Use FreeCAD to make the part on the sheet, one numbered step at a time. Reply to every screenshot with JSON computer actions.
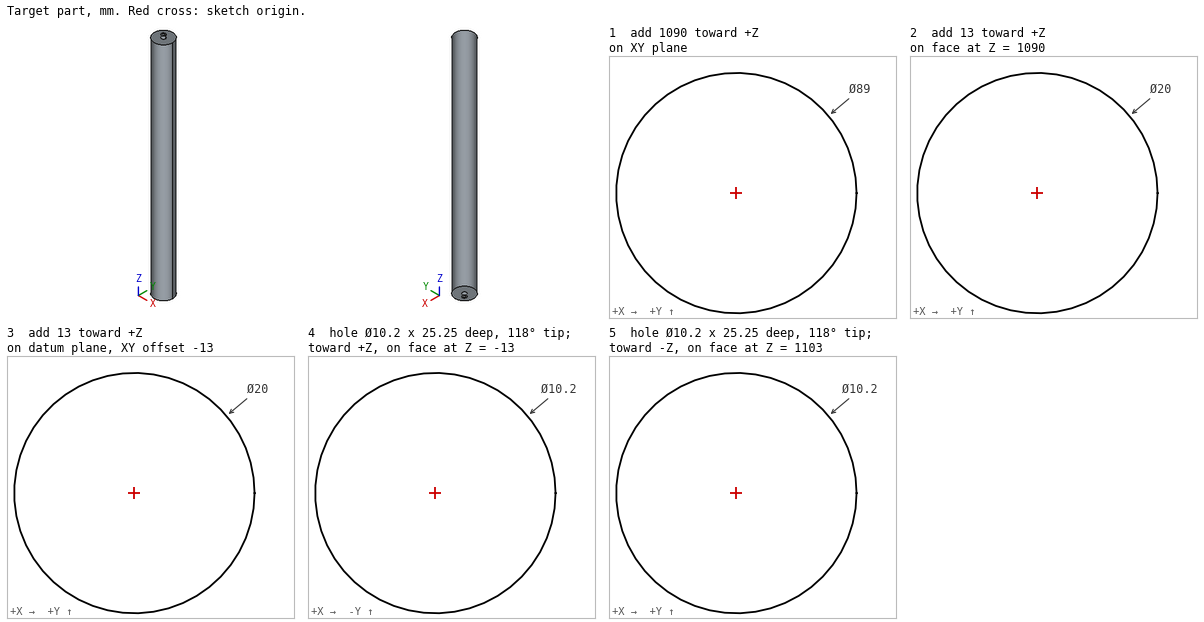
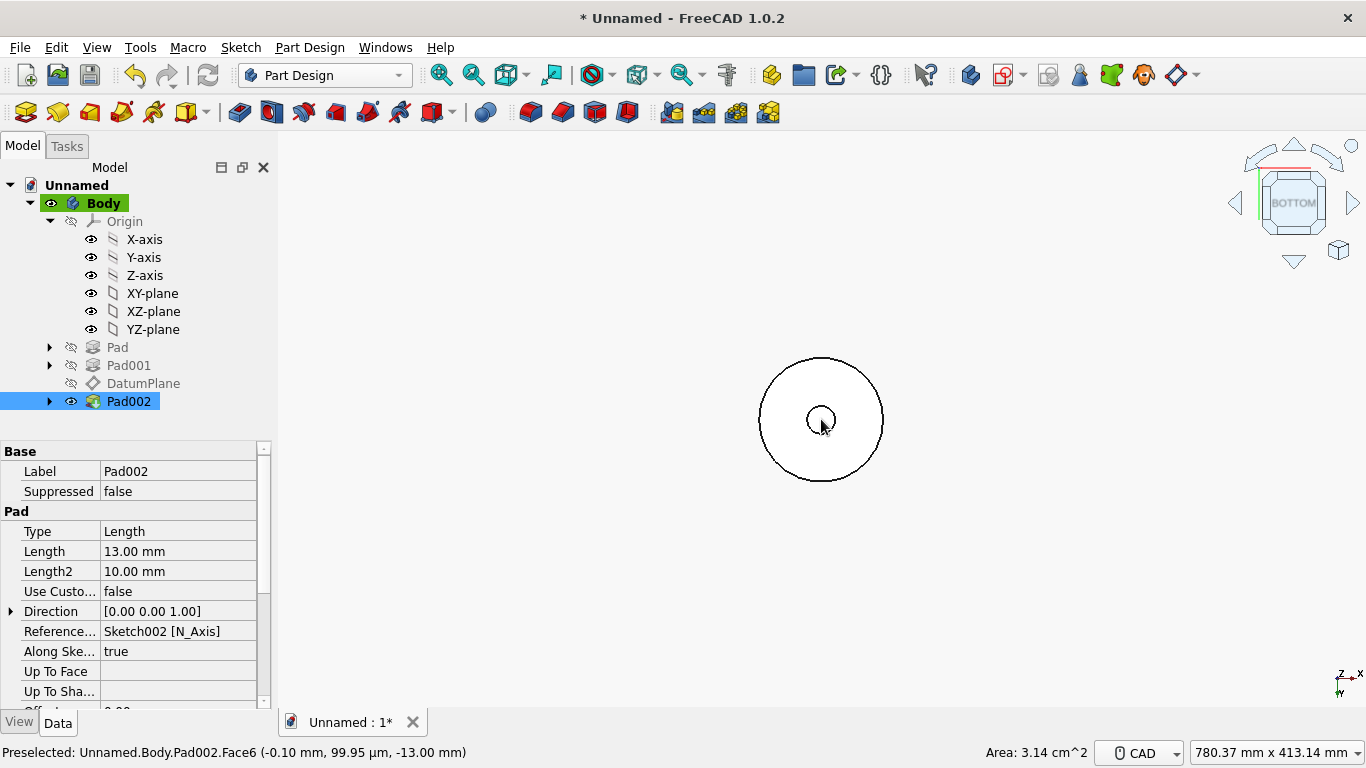
{"action": "left_click", "coordinate": [1004, 76]}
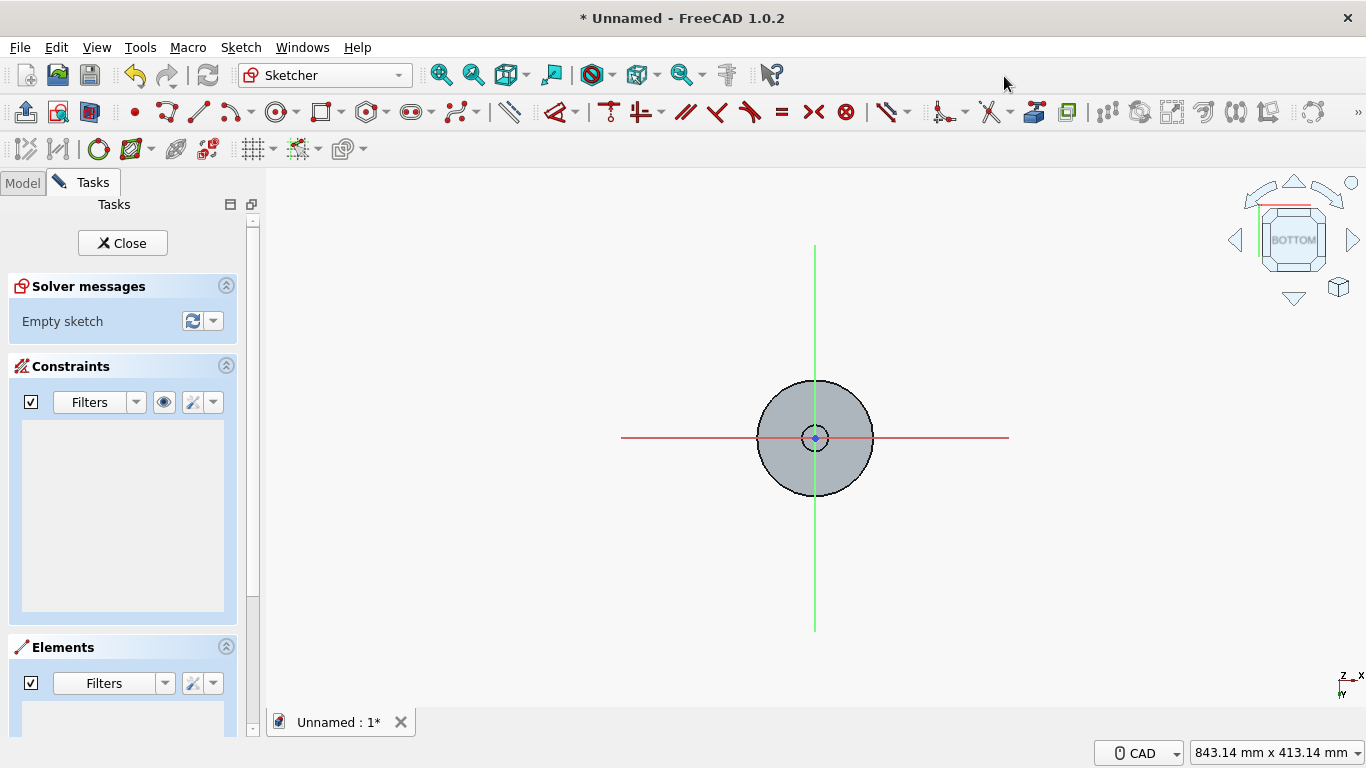
{"action": "scroll", "coordinate": [819, 438], "scroll_direction": "up", "scroll_amount": 15}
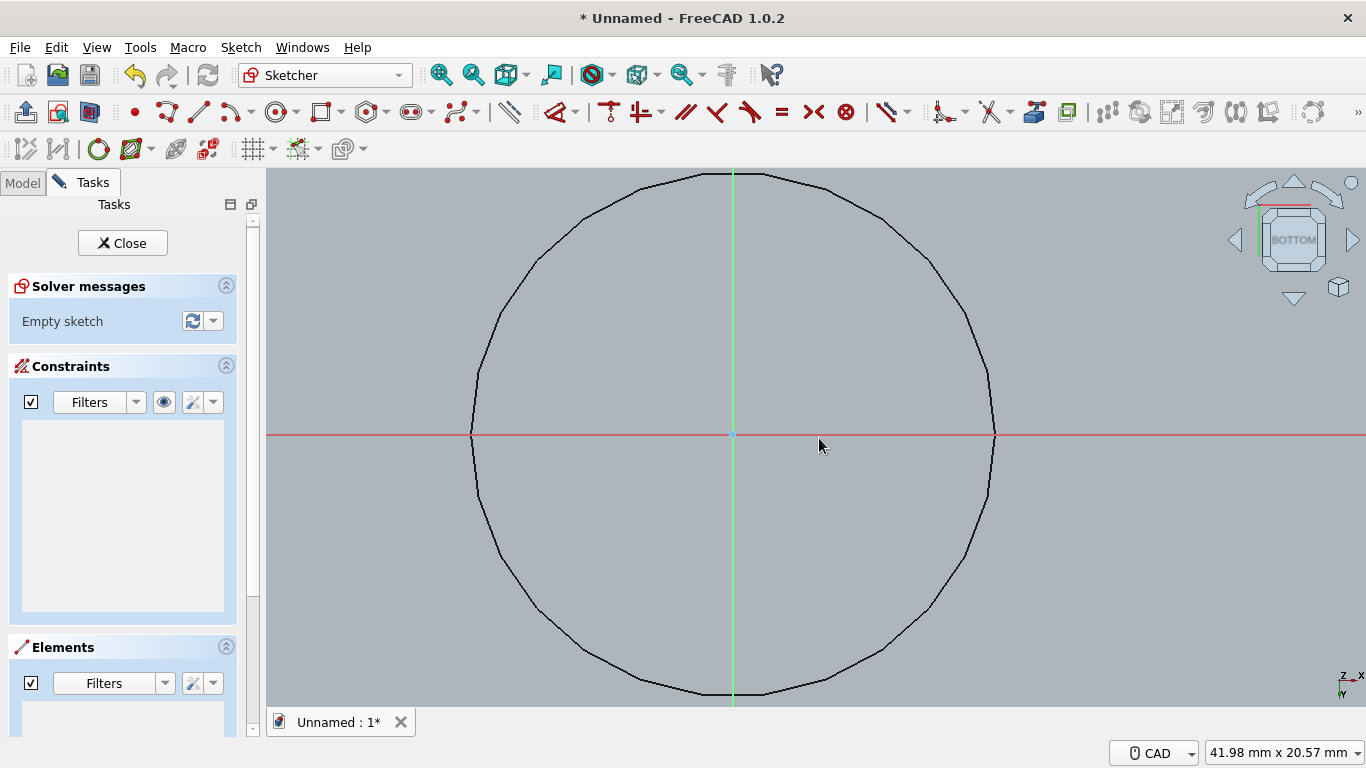
{"action": "key", "text": "g c"}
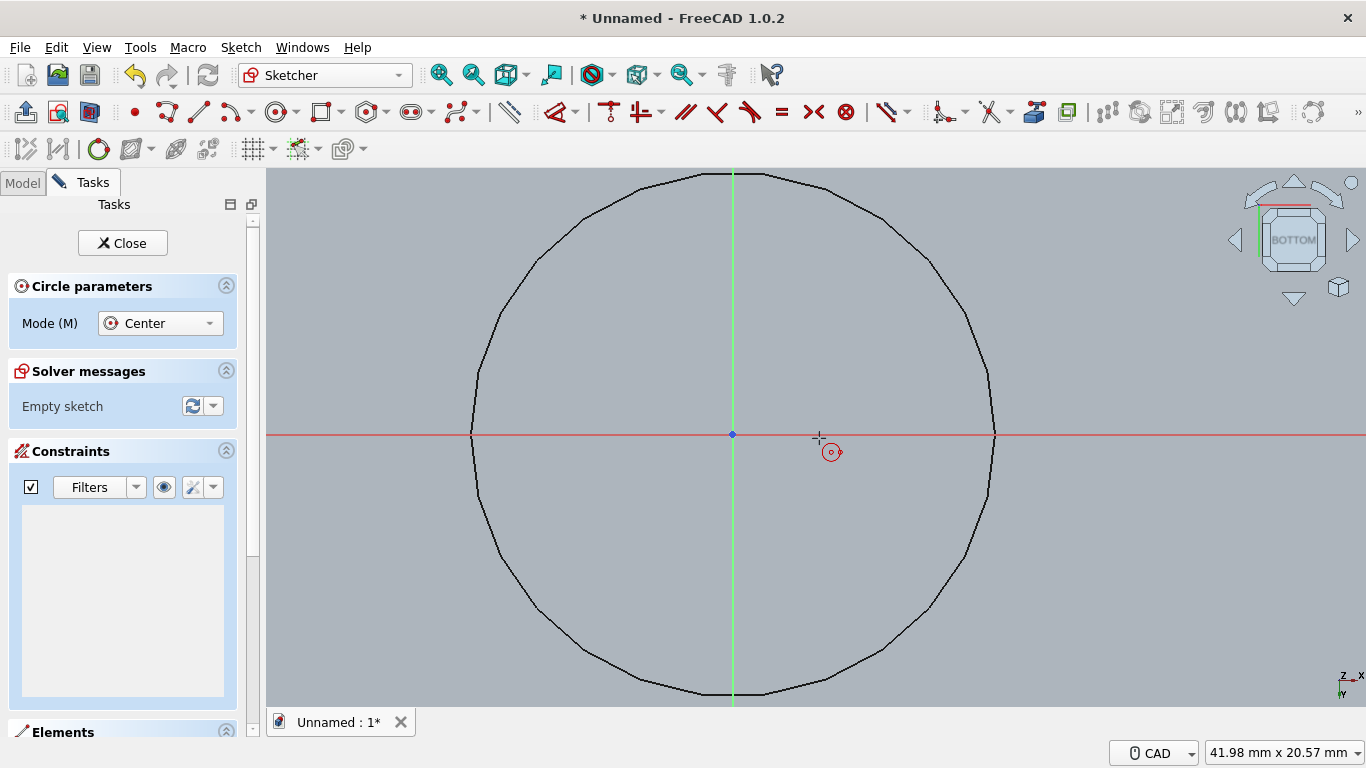
{"action": "left_click", "coordinate": [733, 435]}
{"action": "mouse_move", "coordinate": [827, 340]}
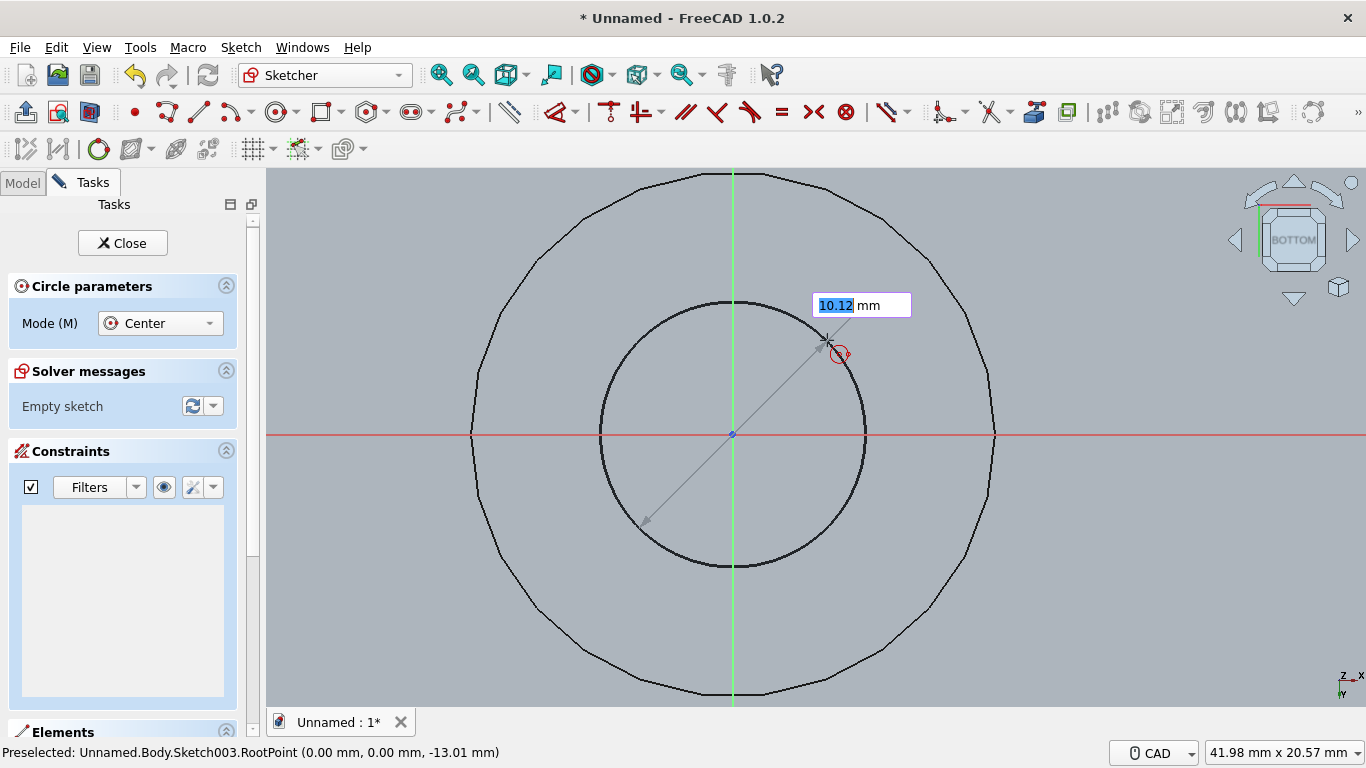
{"action": "type", "text": "10.2"}
{"action": "key", "text": "Return"}
{"action": "key", "text": "Escape"}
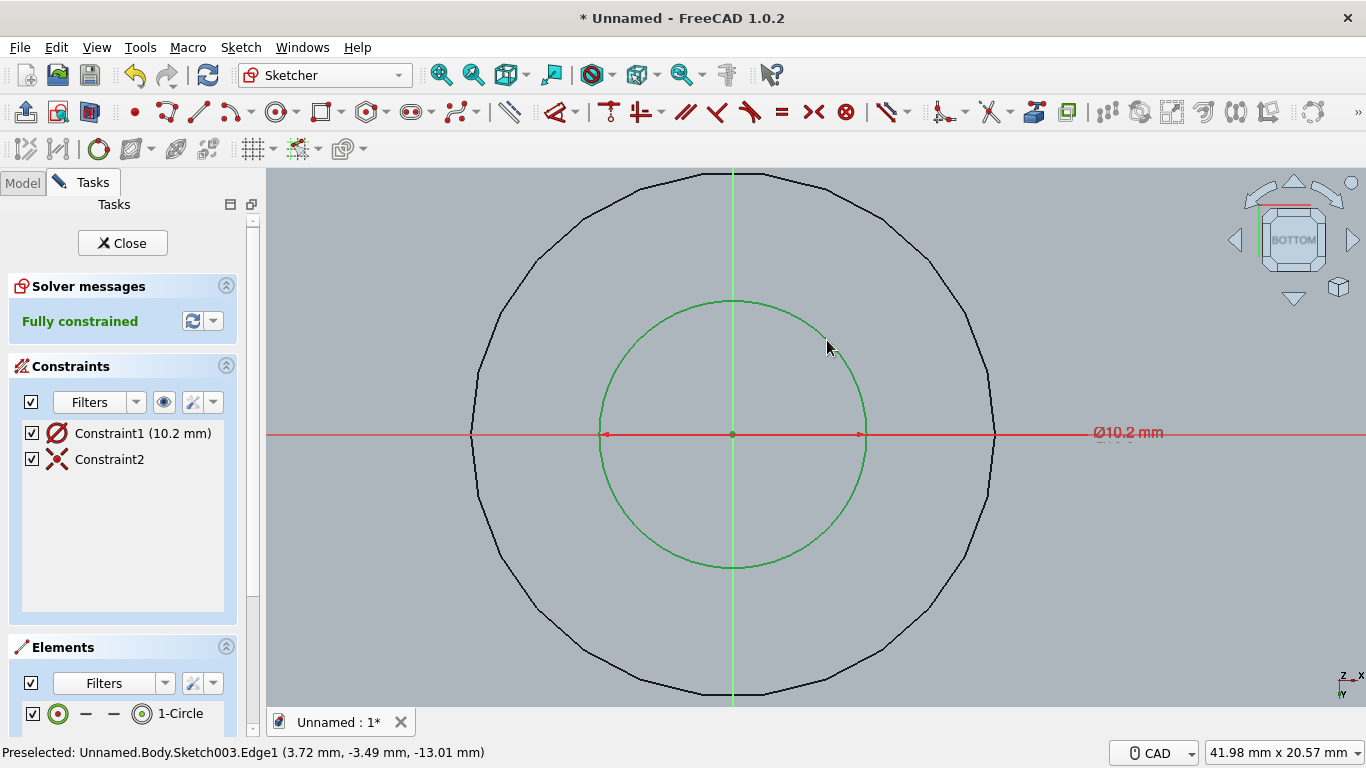
{"action": "left_click", "coordinate": [123, 243]}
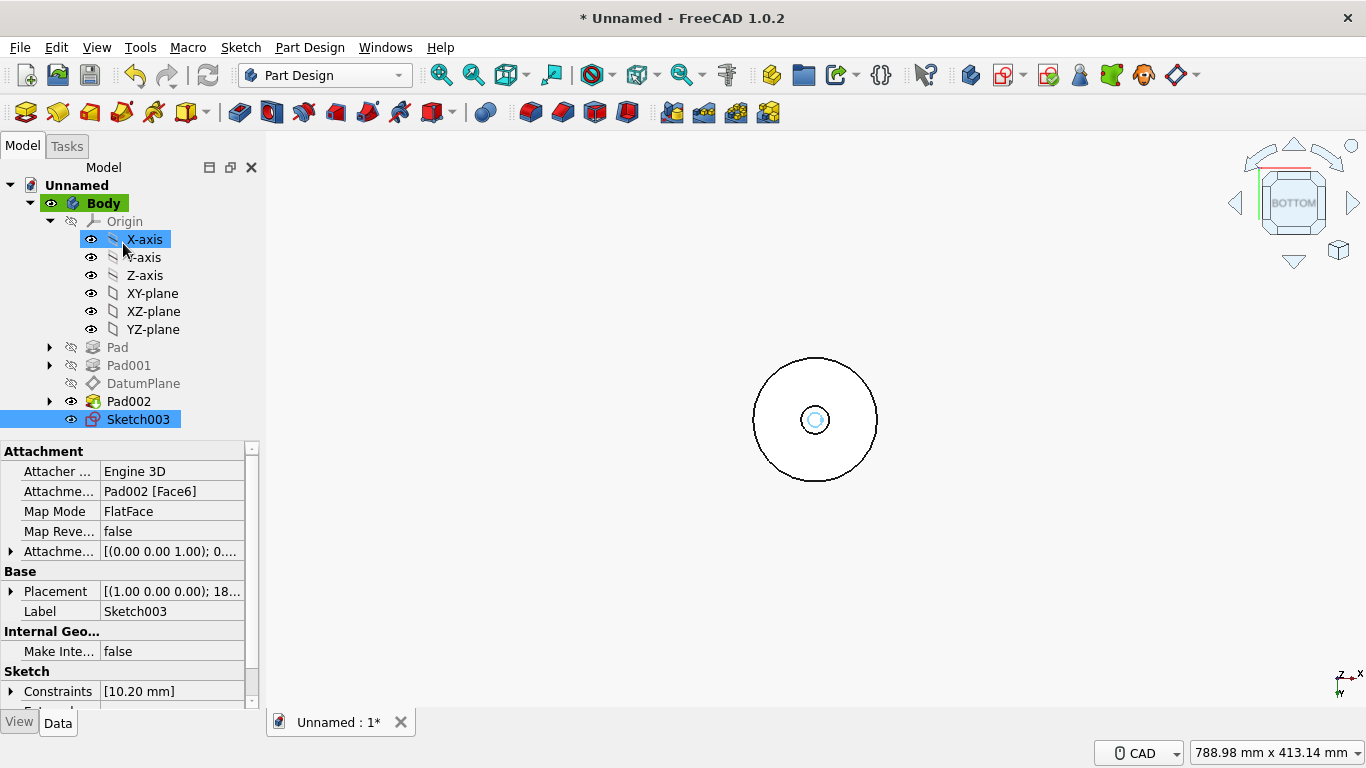
{"action": "left_click", "coordinate": [272, 112]}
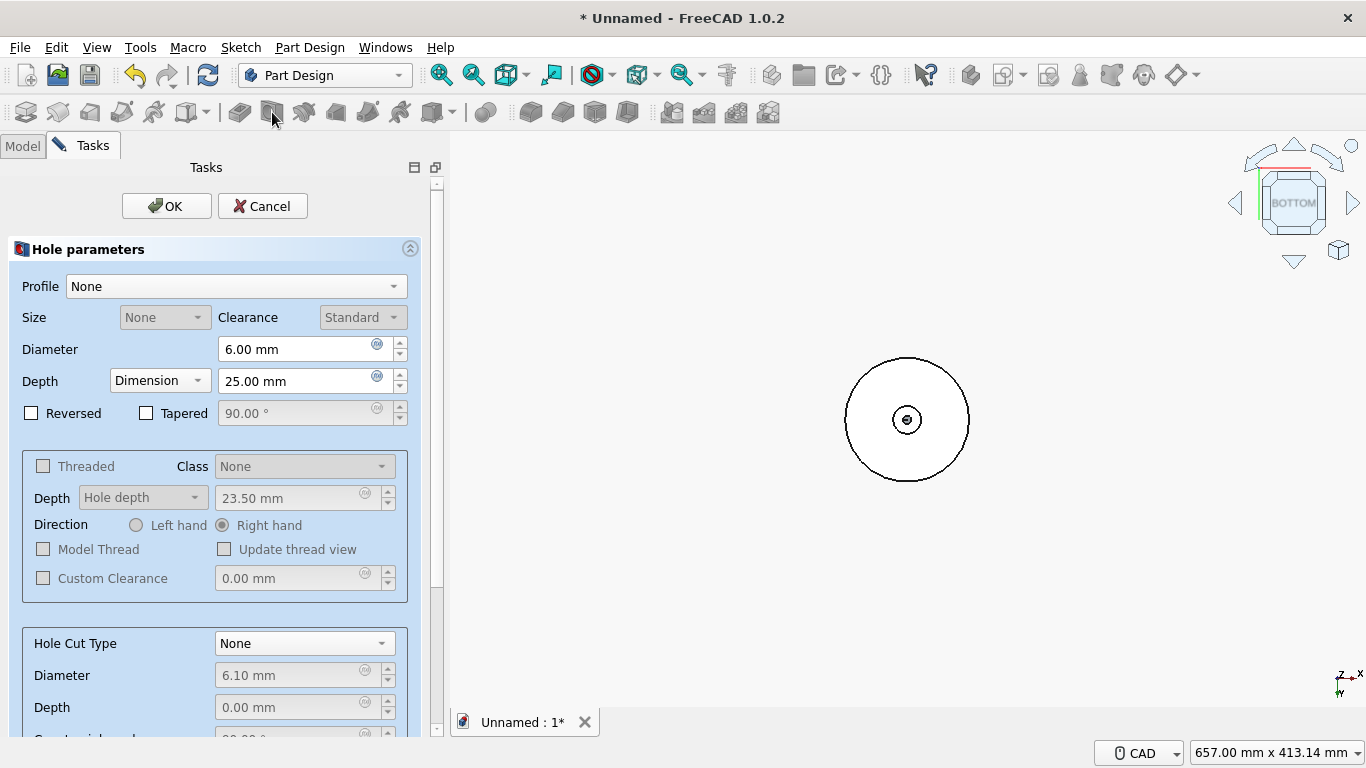
{"action": "triple_click", "coordinate": [305, 349]}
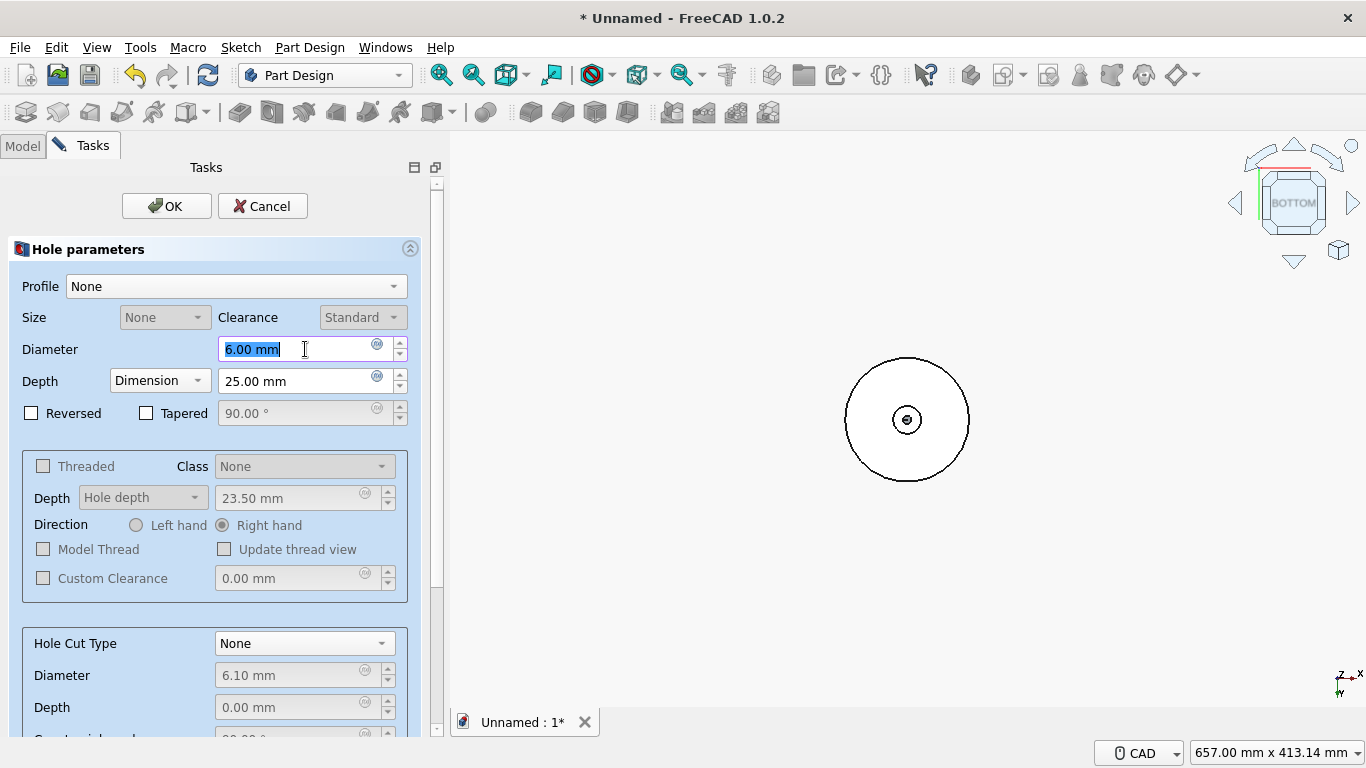
{"action": "type", "text": "10.2"}
{"action": "key", "text": "Tab"}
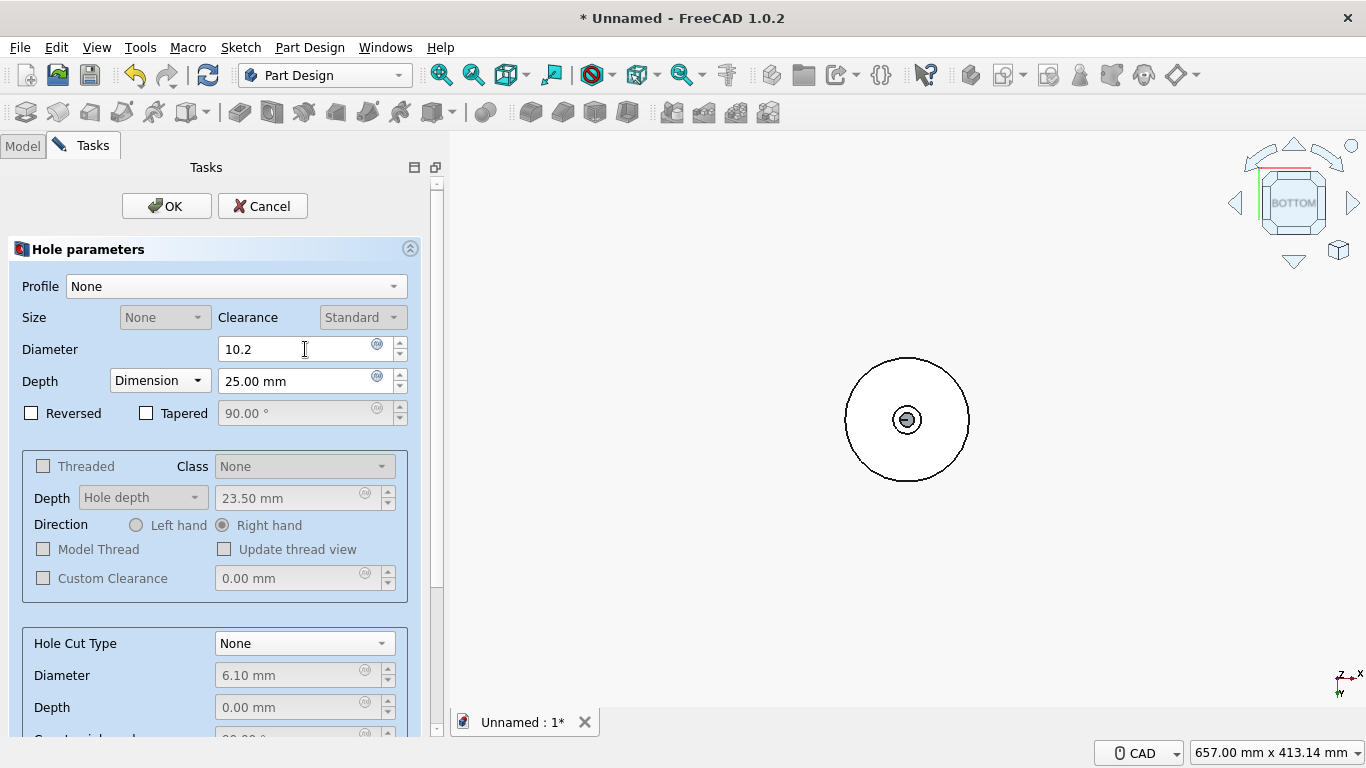
{"action": "triple_click", "coordinate": [305, 381]}